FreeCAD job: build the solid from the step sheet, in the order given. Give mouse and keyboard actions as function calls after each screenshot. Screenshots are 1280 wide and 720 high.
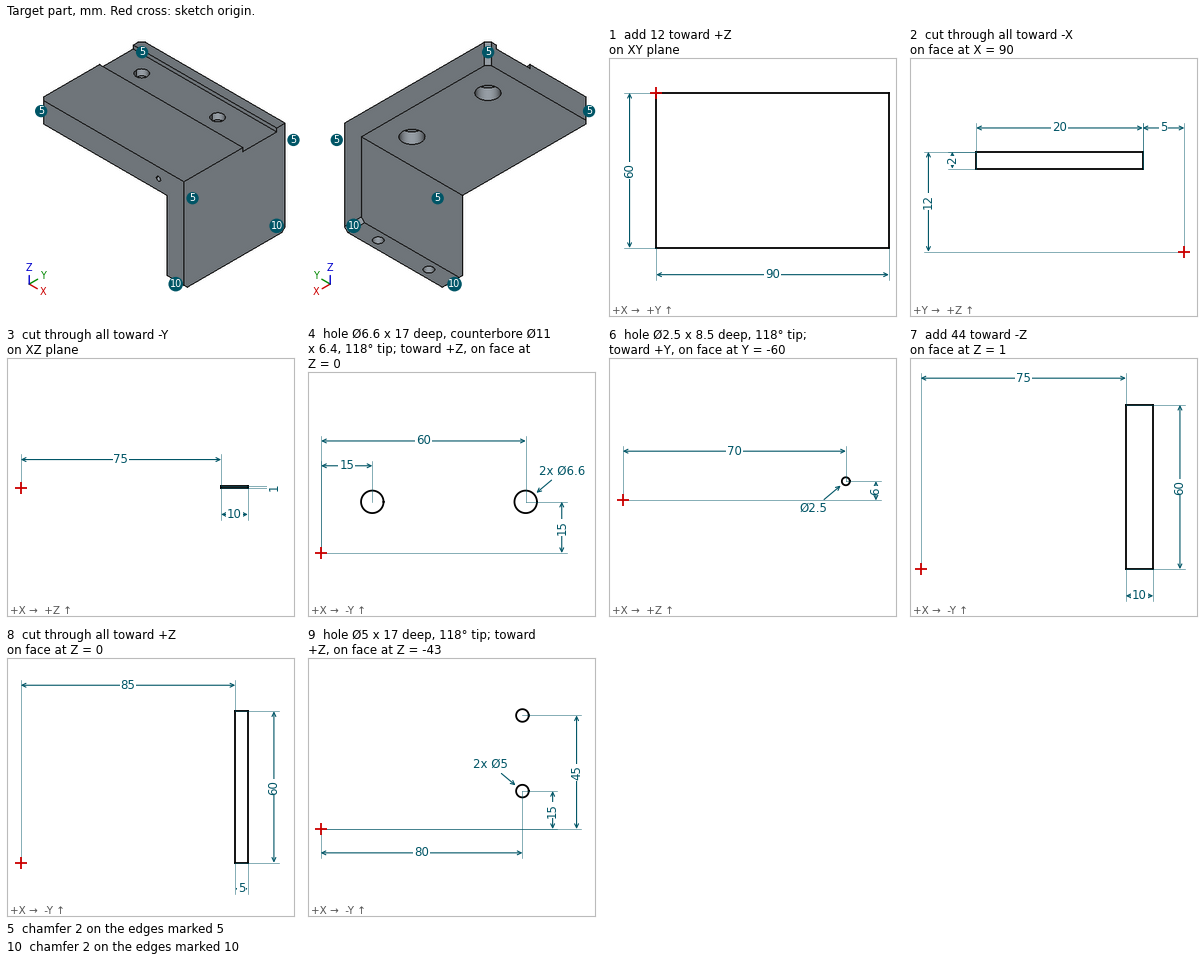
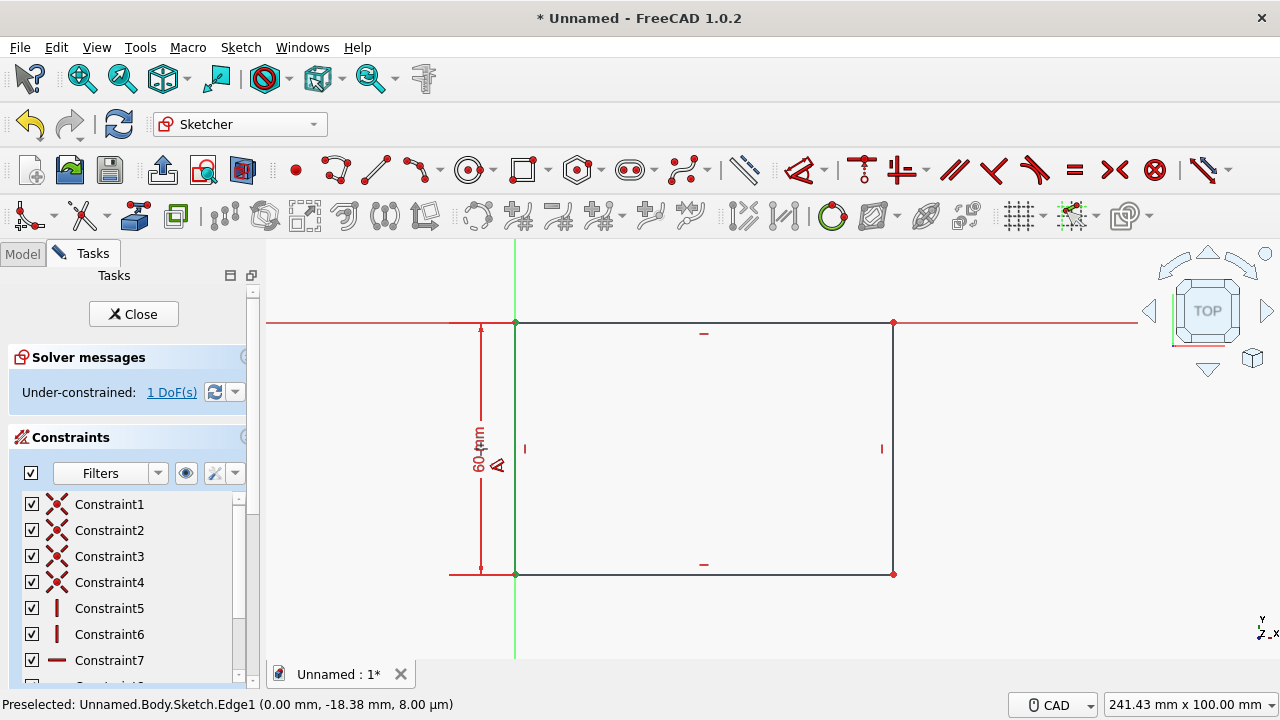
click(628, 575)
click(704, 609)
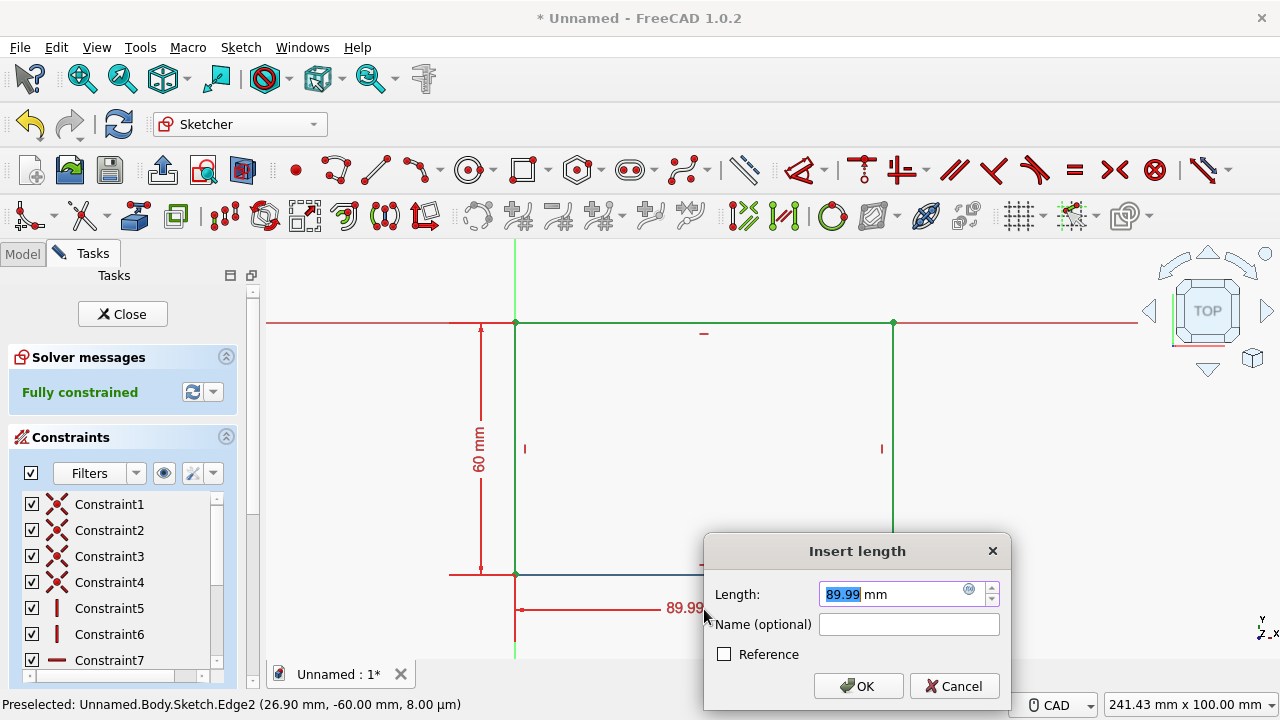
text(90)
key(Return)
key(Escape)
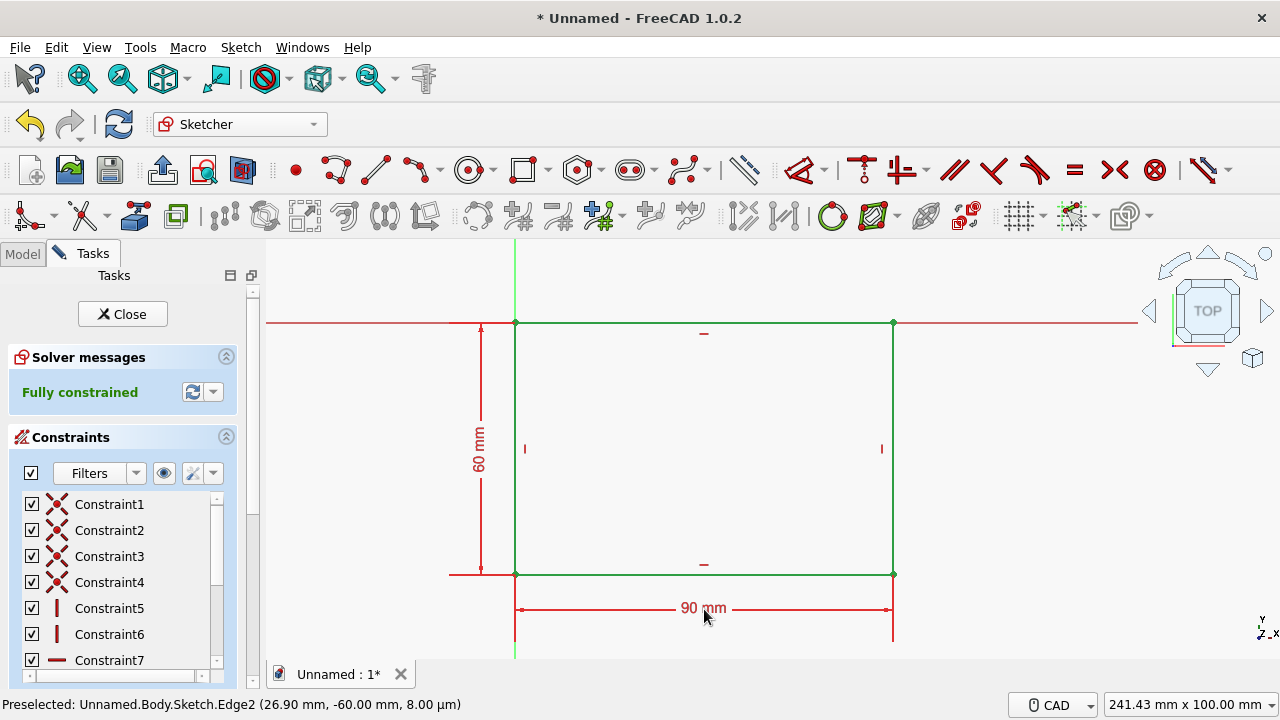
click(123, 314)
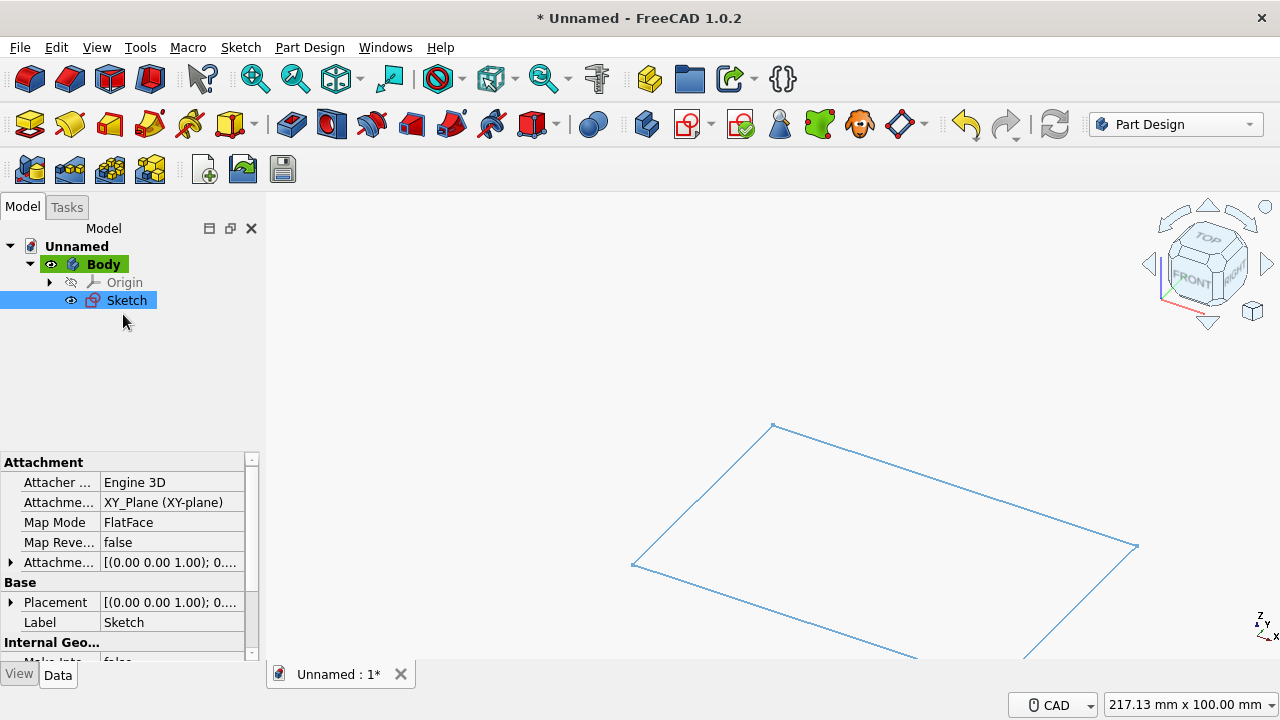
click(30, 124)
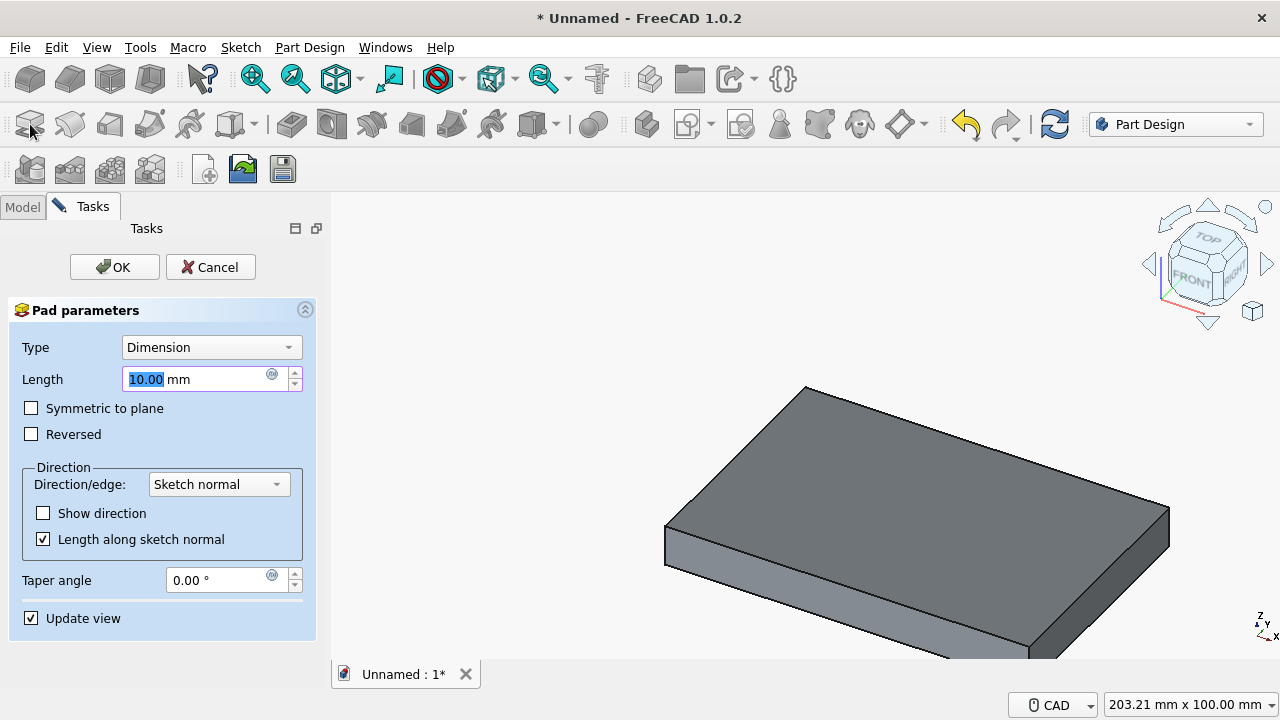
text(12)
key(Tab)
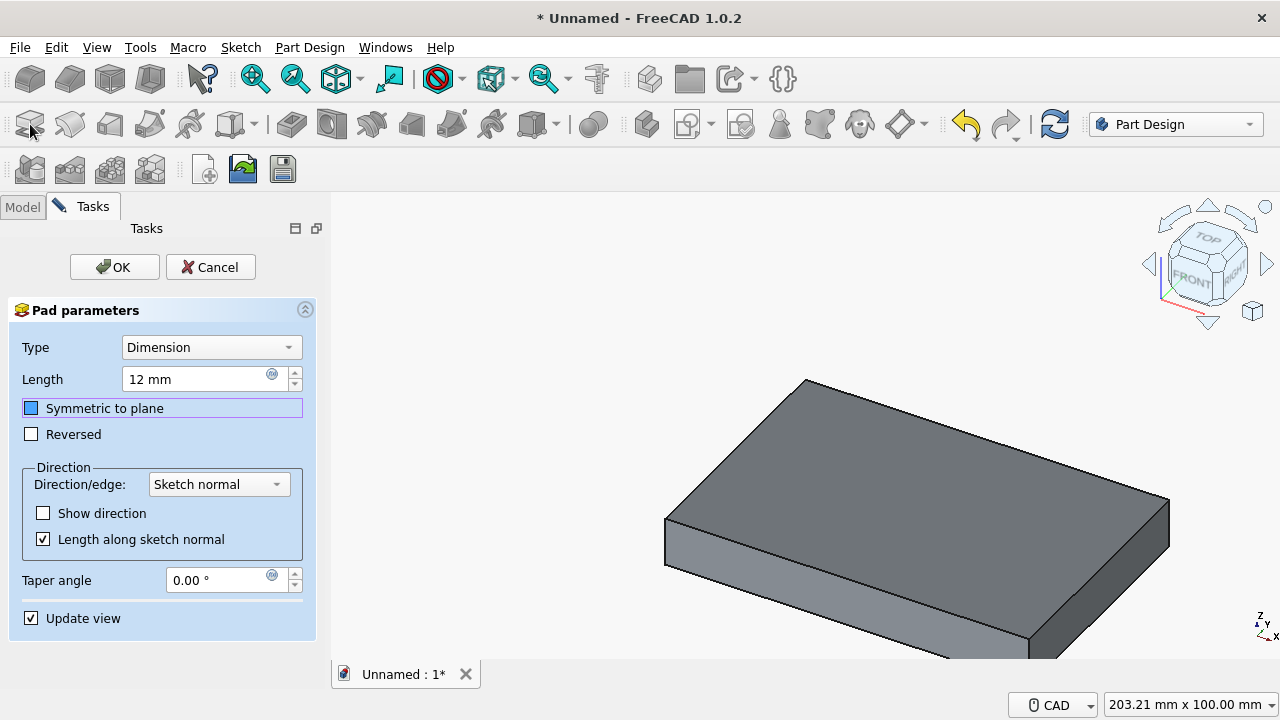
click(115, 267)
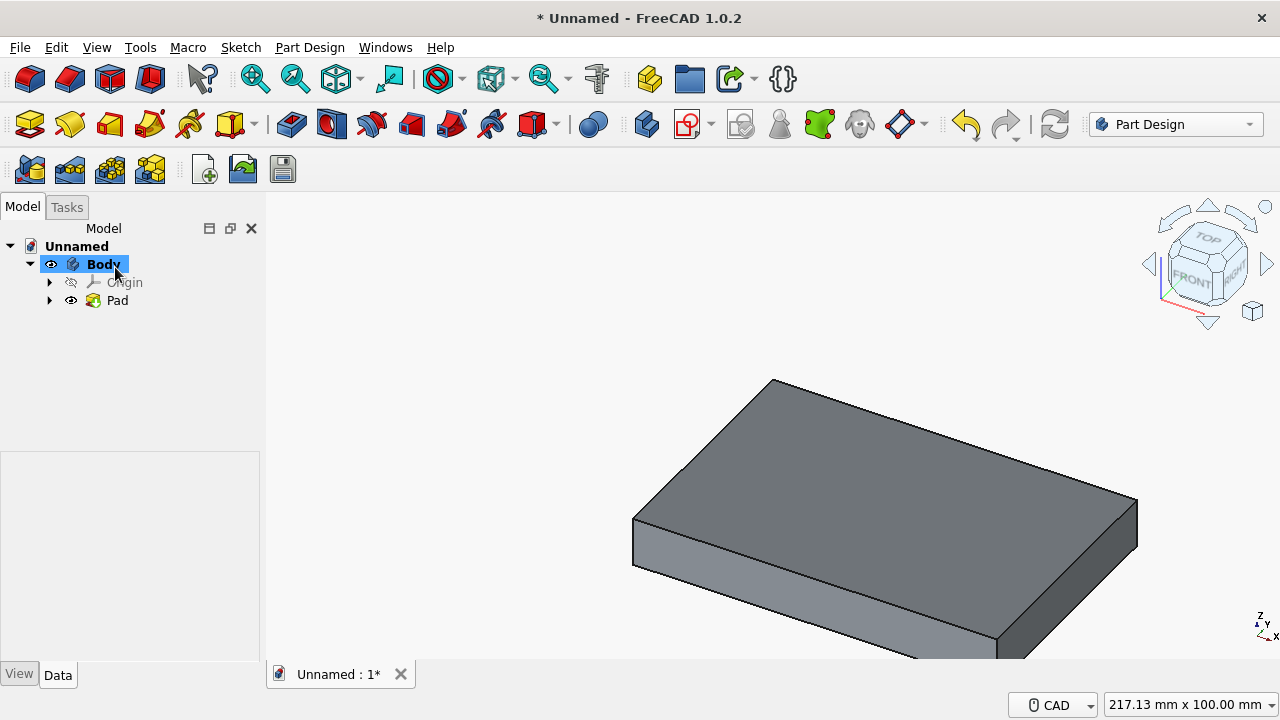
click(256, 80)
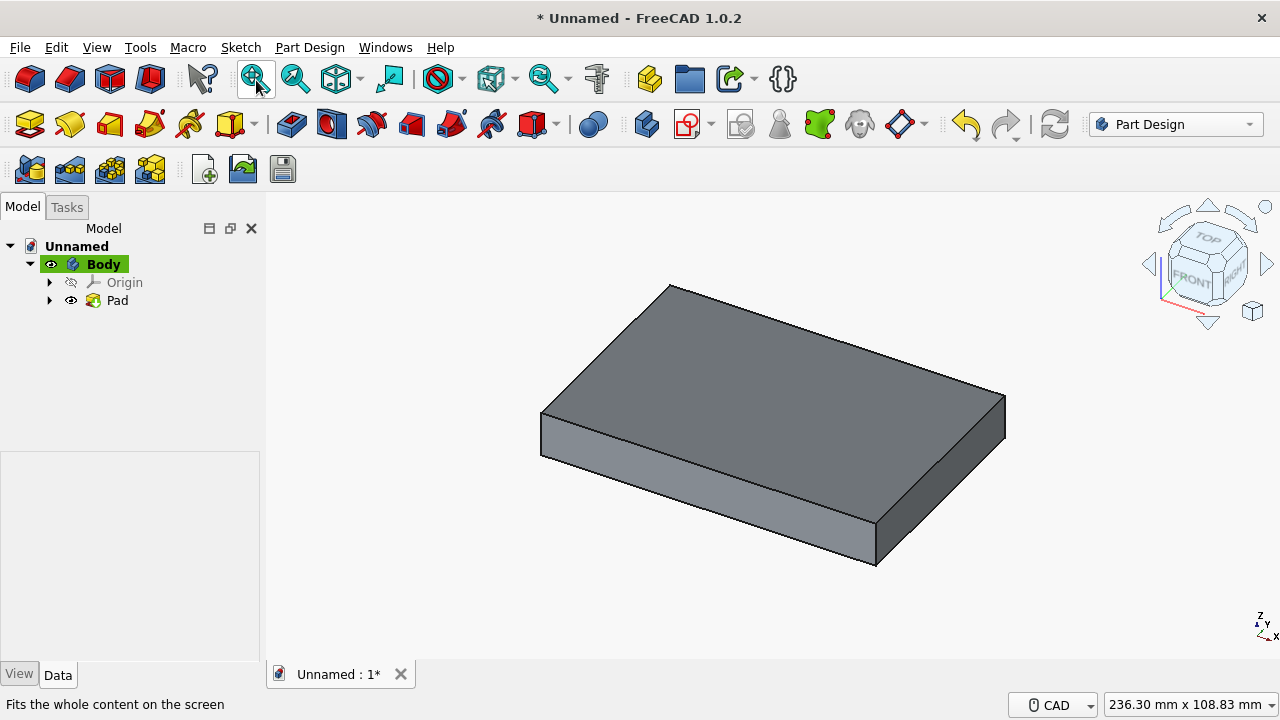
click(977, 443)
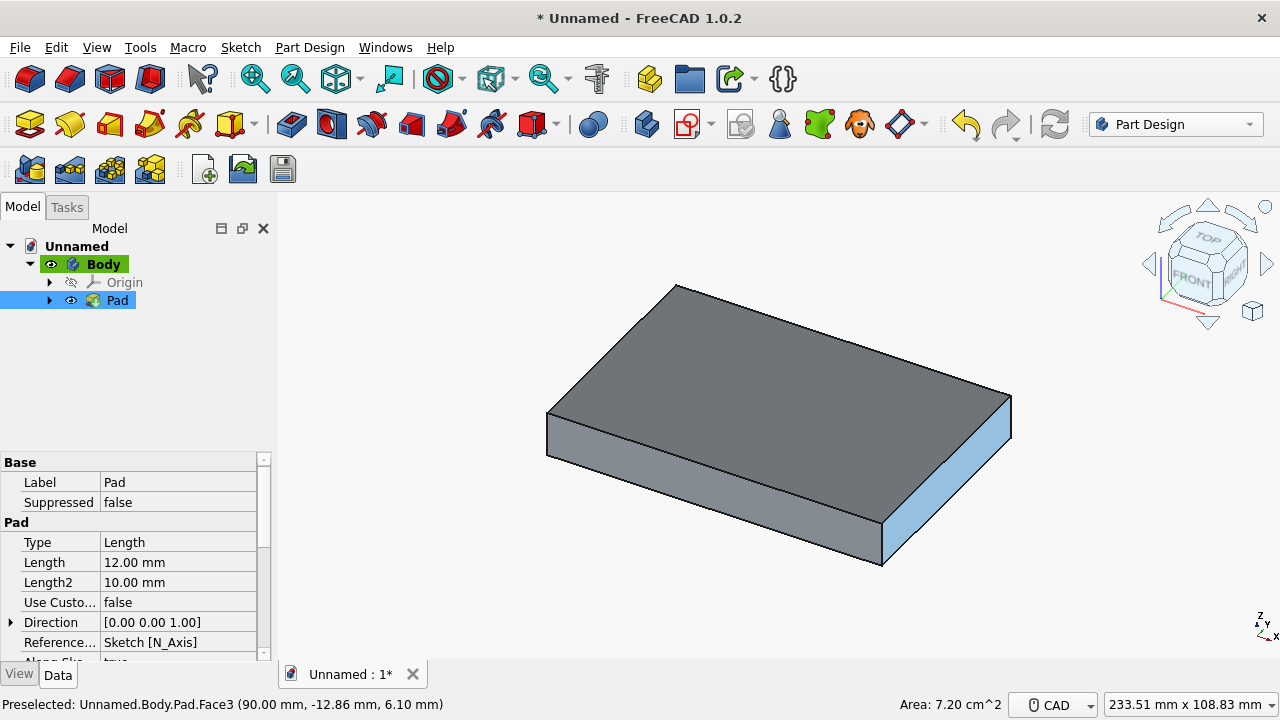
click(688, 124)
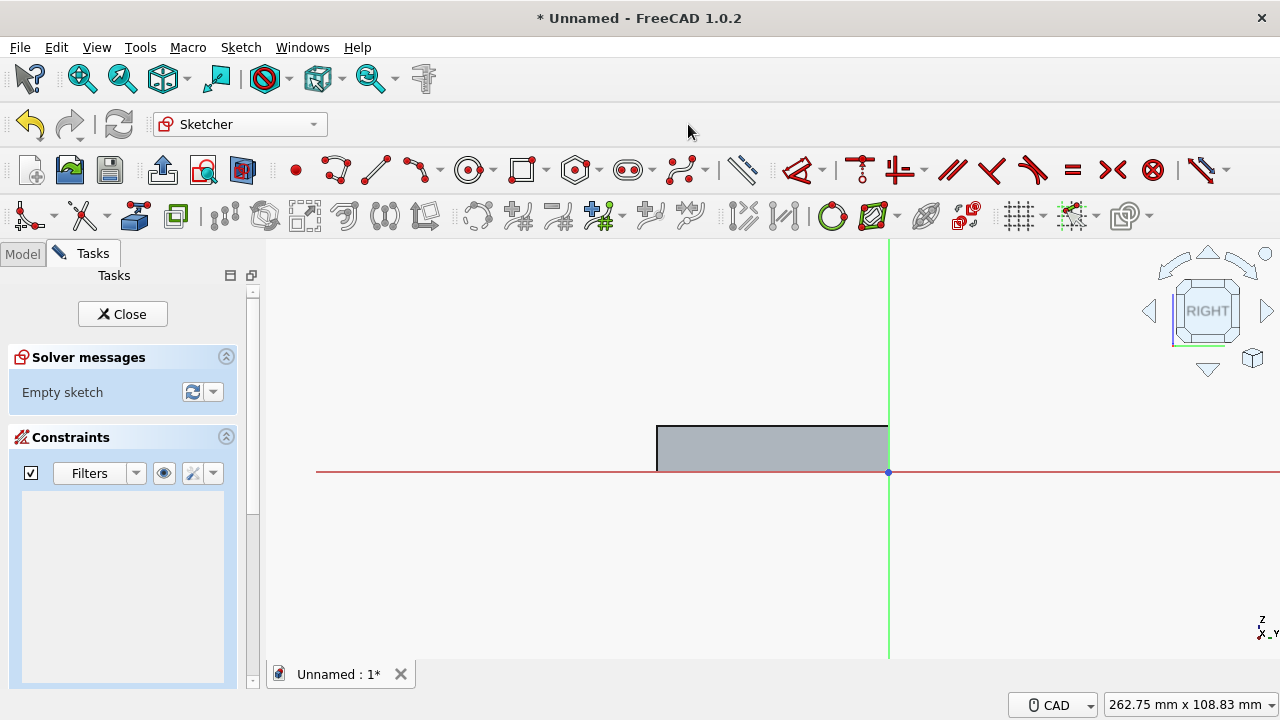
scroll(867, 449, up, 9)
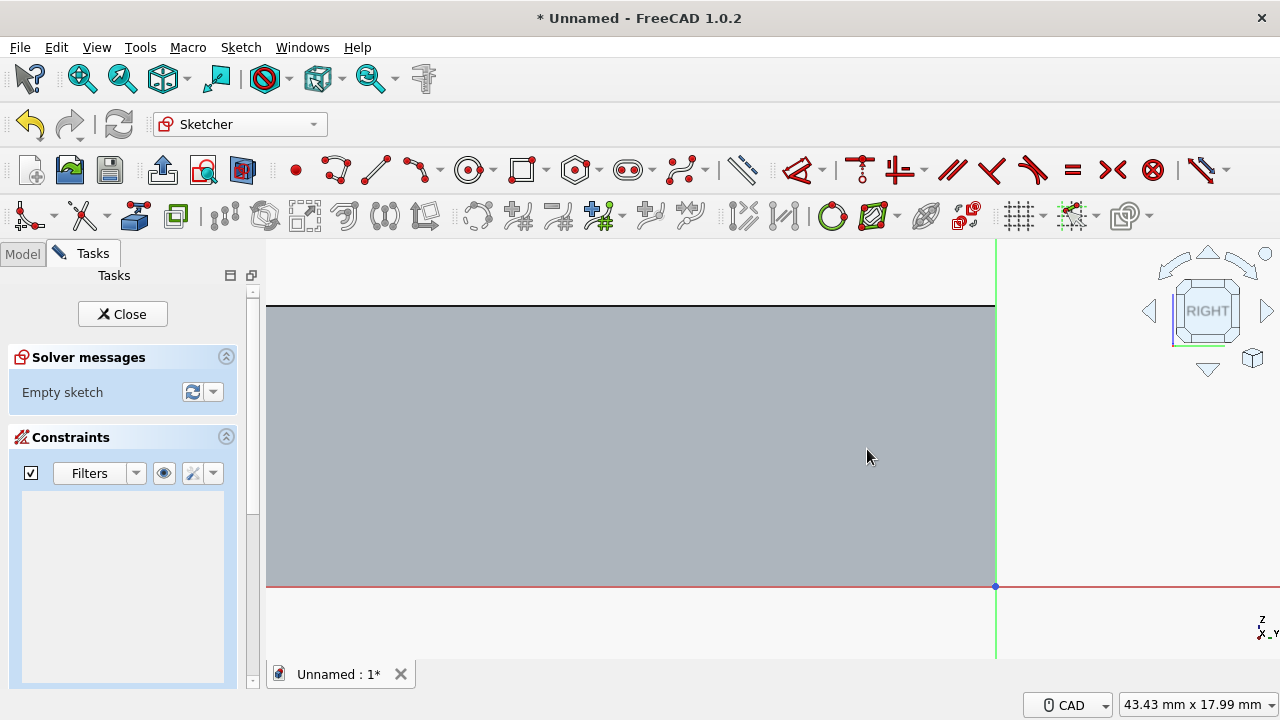
click(522, 170)